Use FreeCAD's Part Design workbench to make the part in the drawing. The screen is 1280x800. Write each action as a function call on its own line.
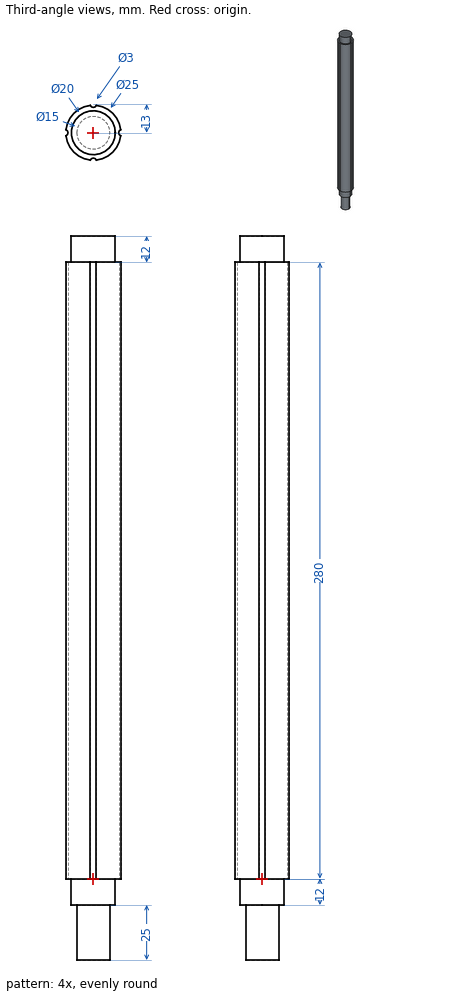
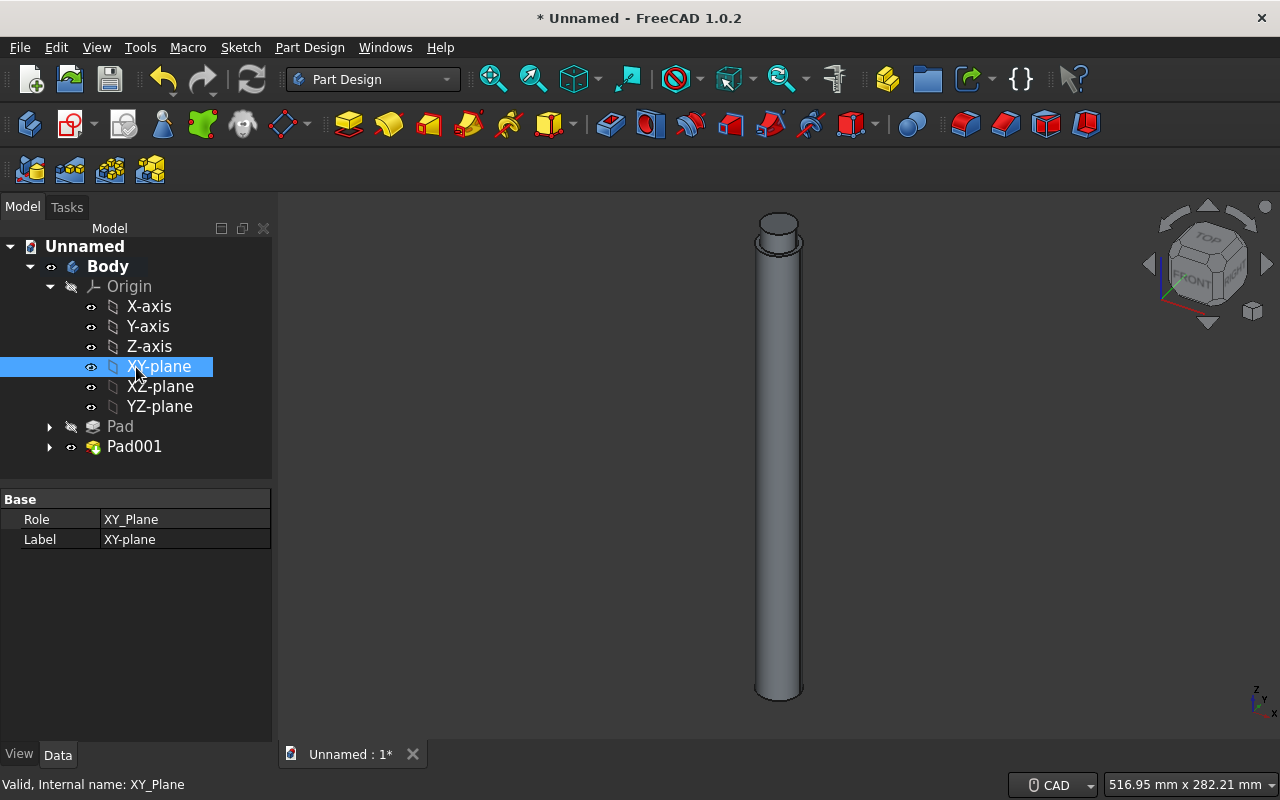
click(284, 124)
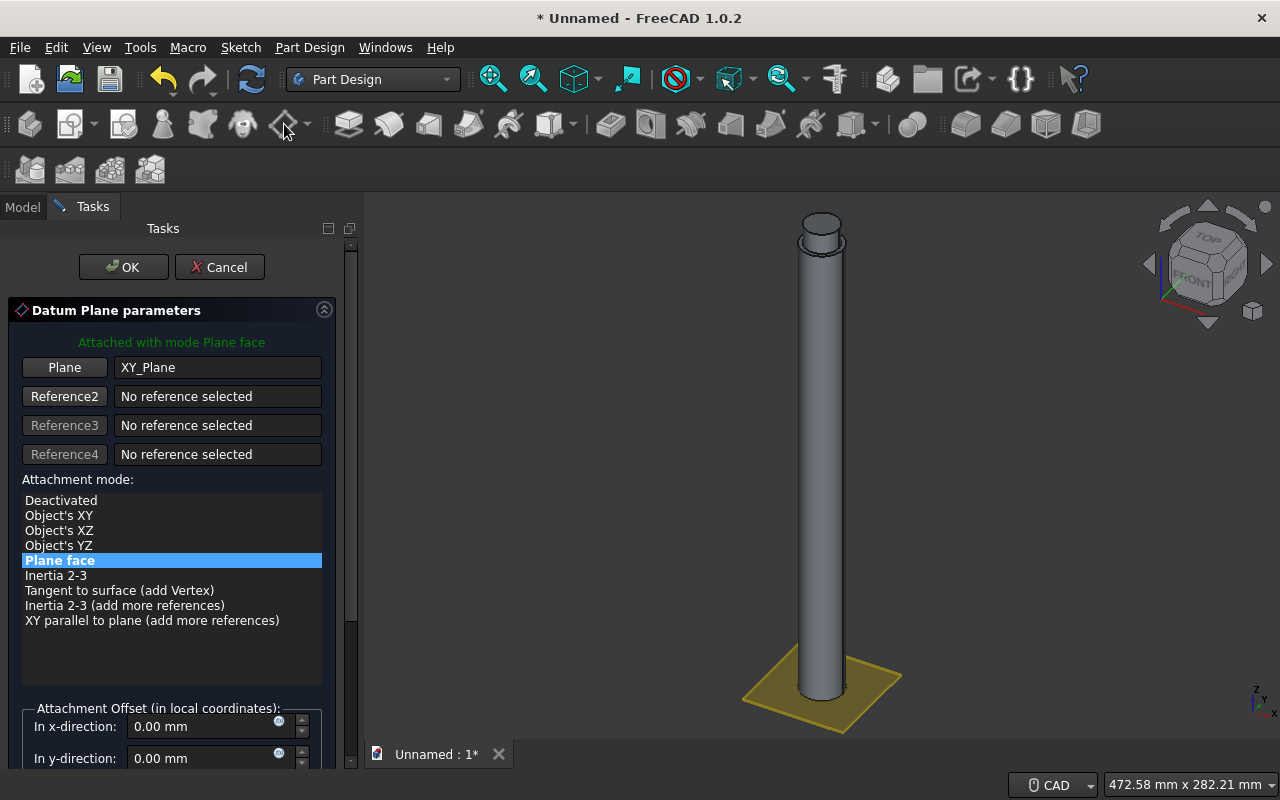
scroll(351, 503, down, 2)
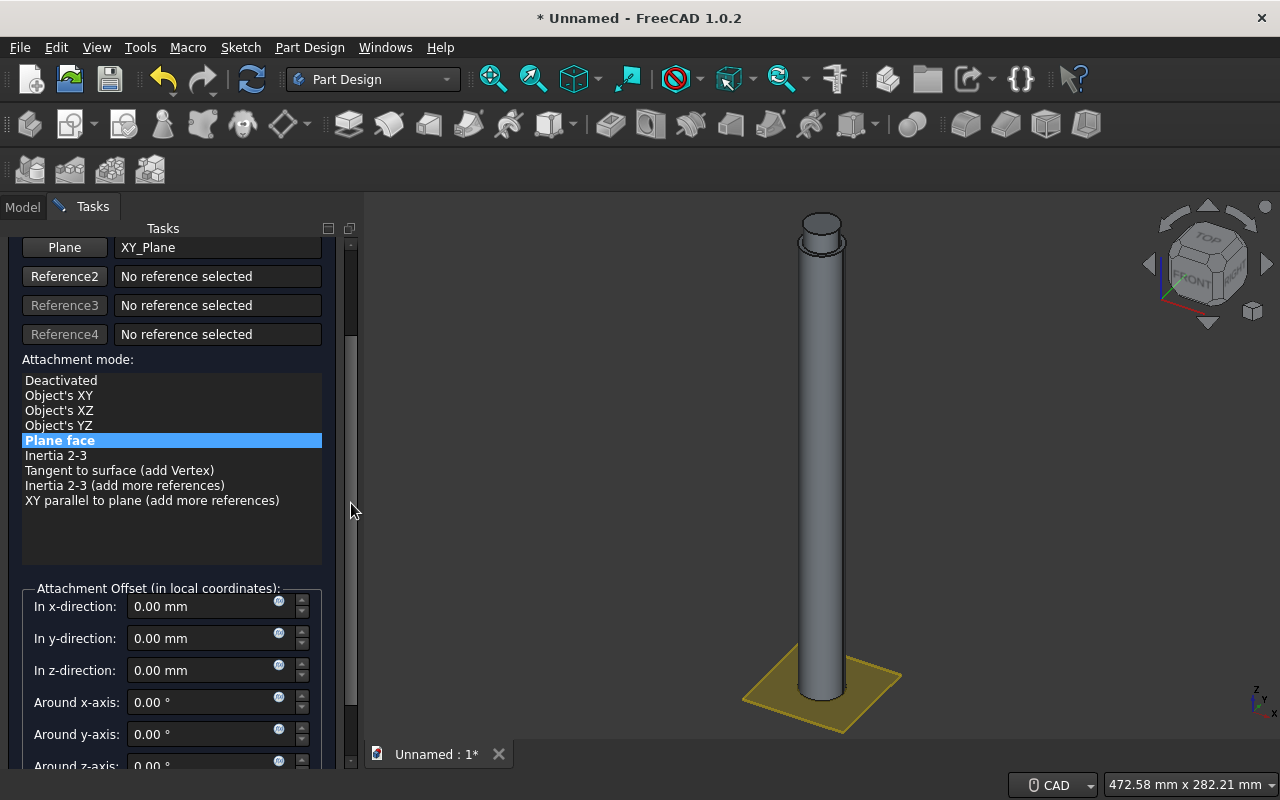
triple_click(210, 670)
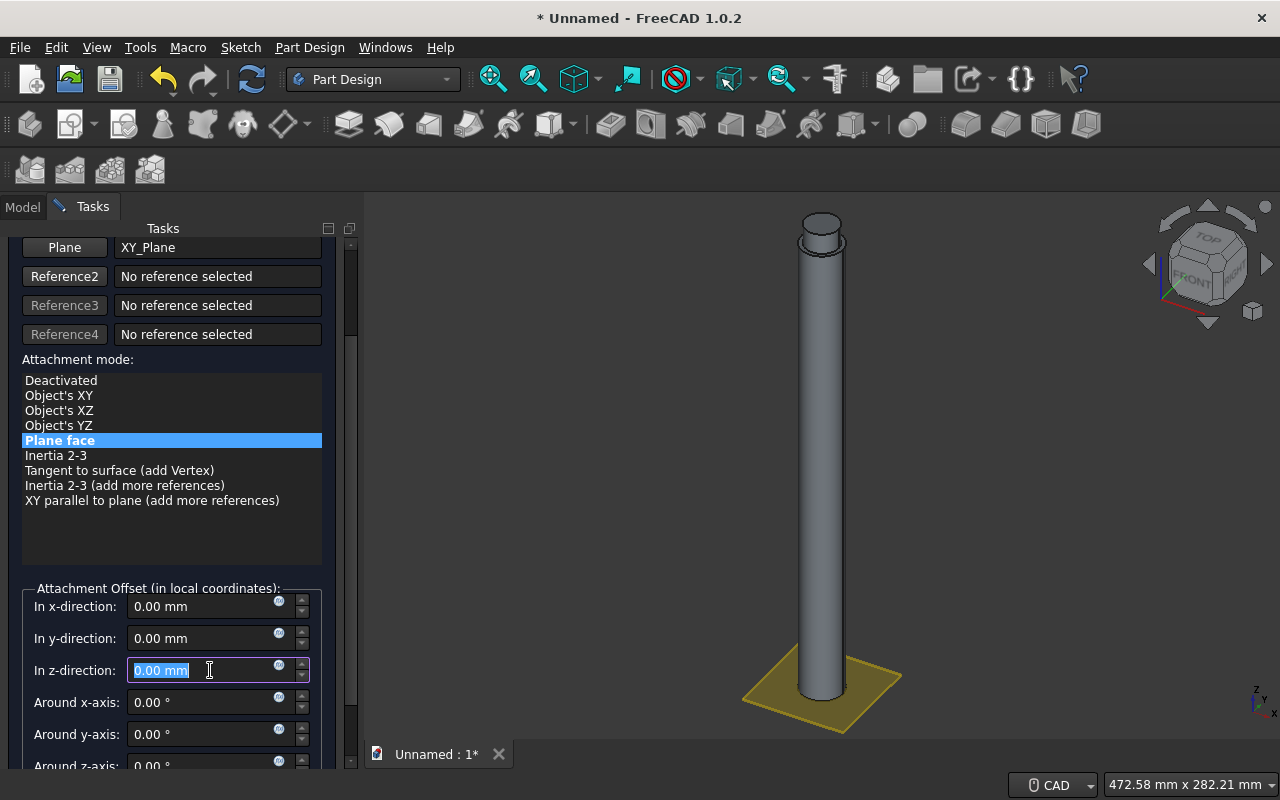
text(-12)
key(Tab)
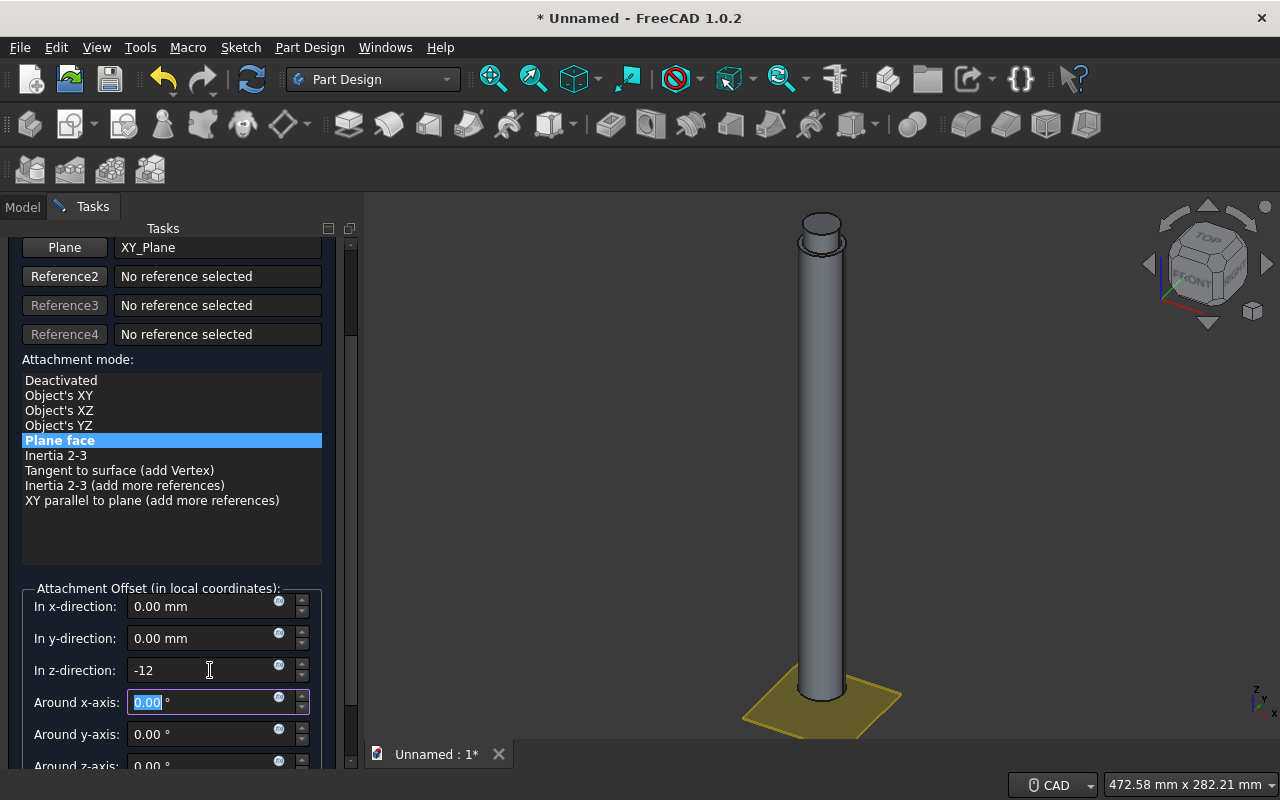
scroll(351, 503, up, 3)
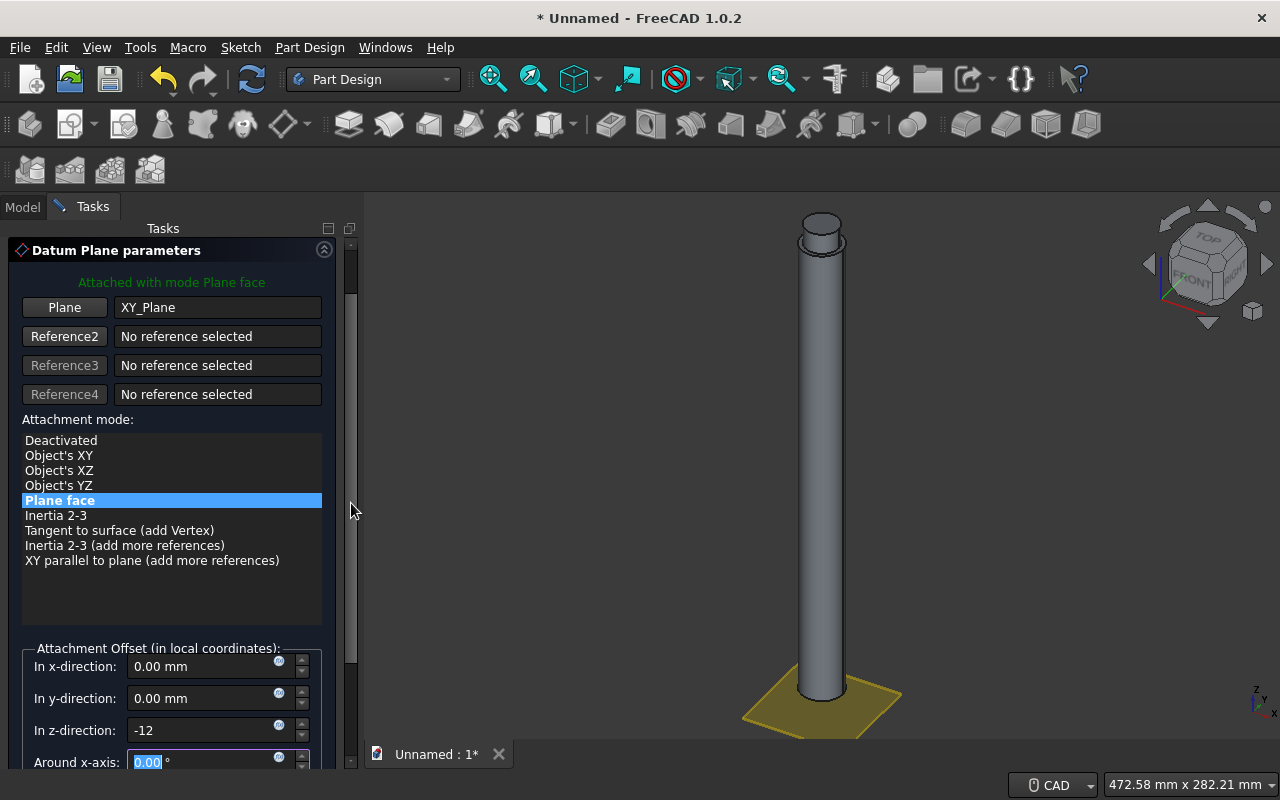
click(124, 267)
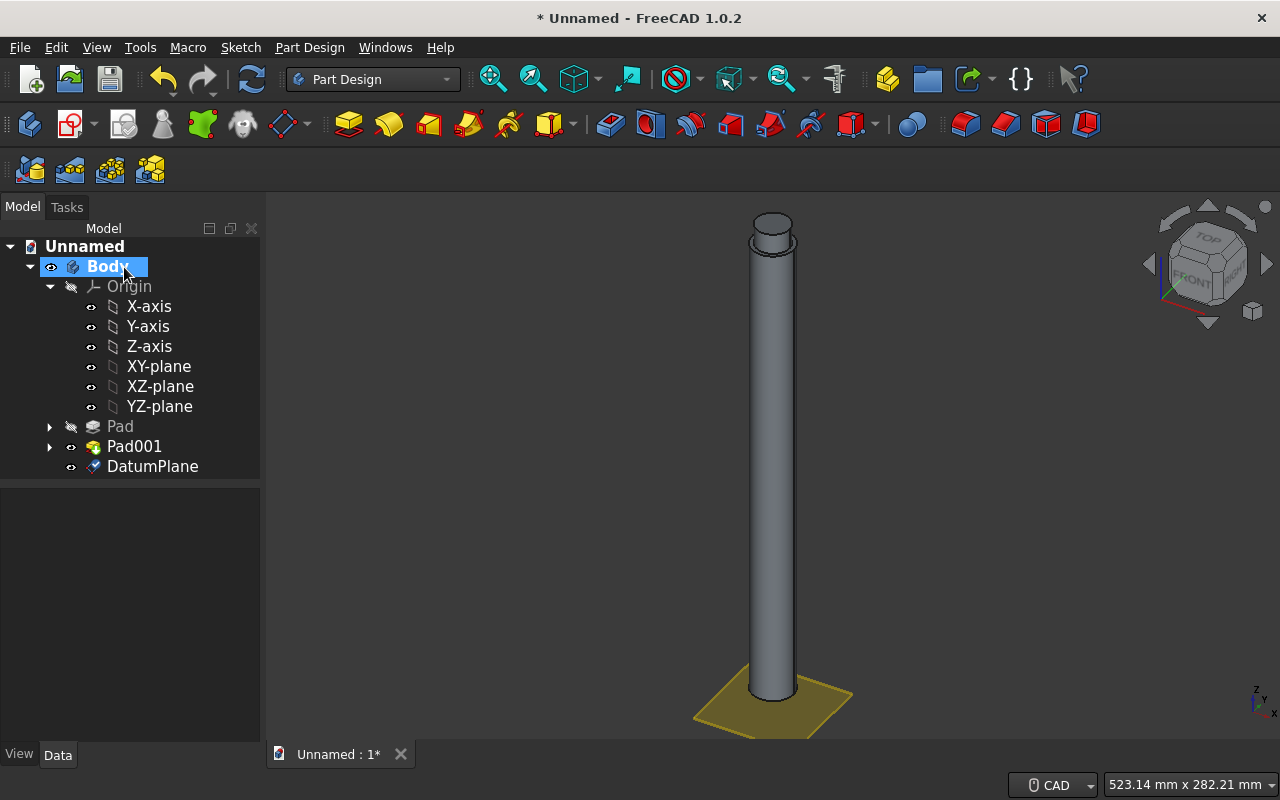
click(116, 467)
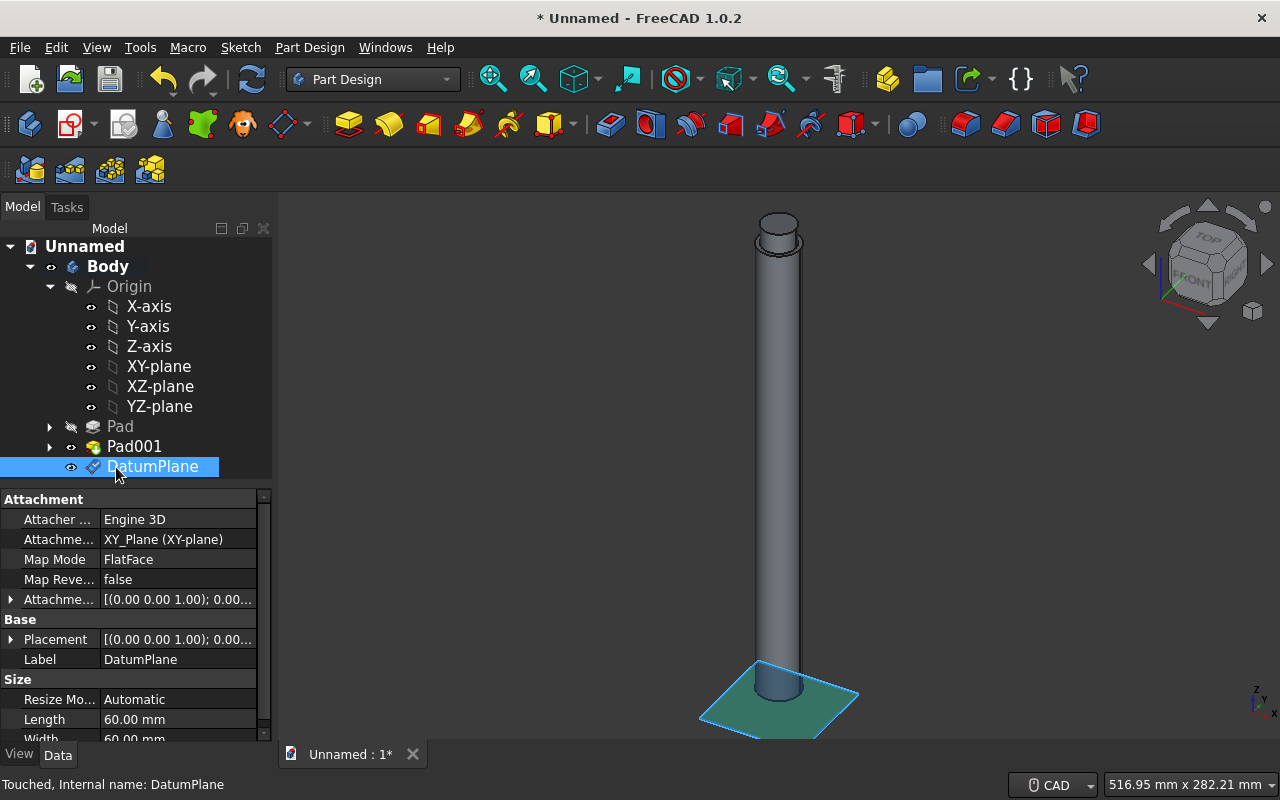
click(70, 124)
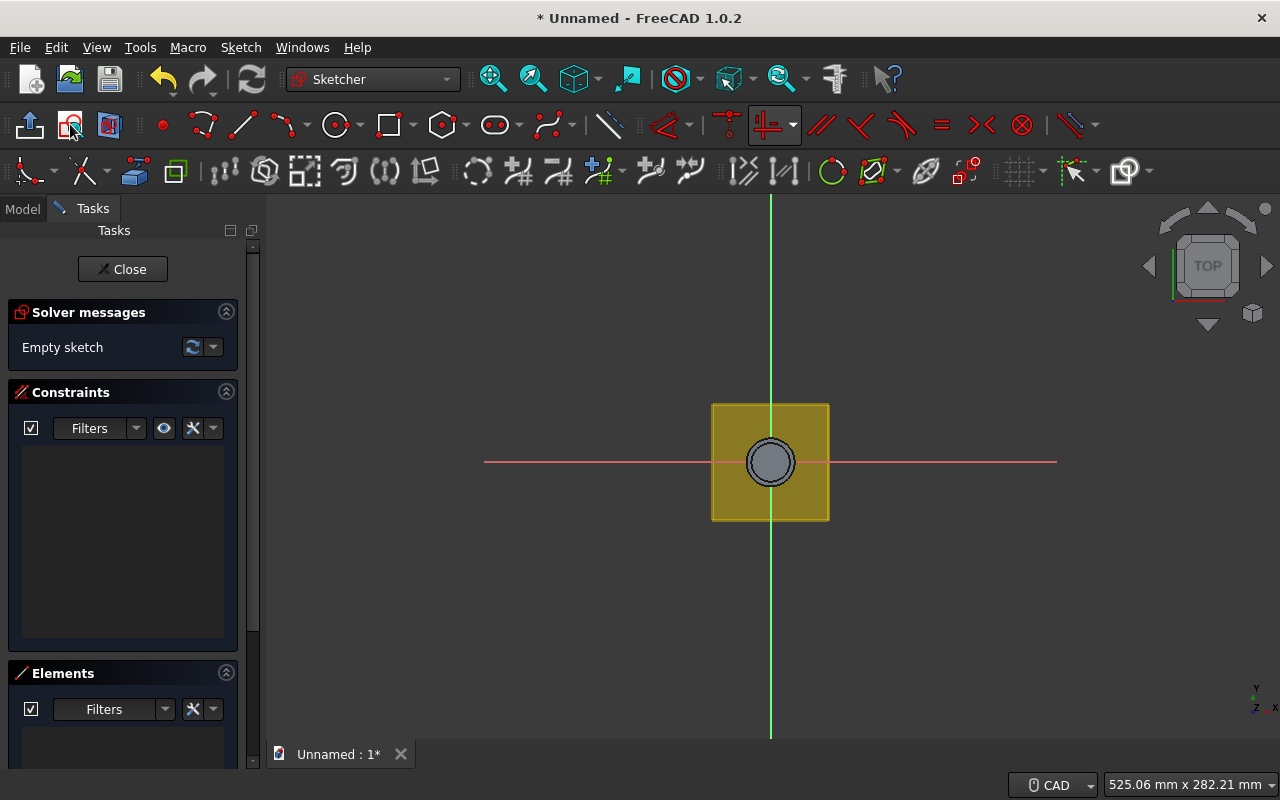
key(q)
key(s)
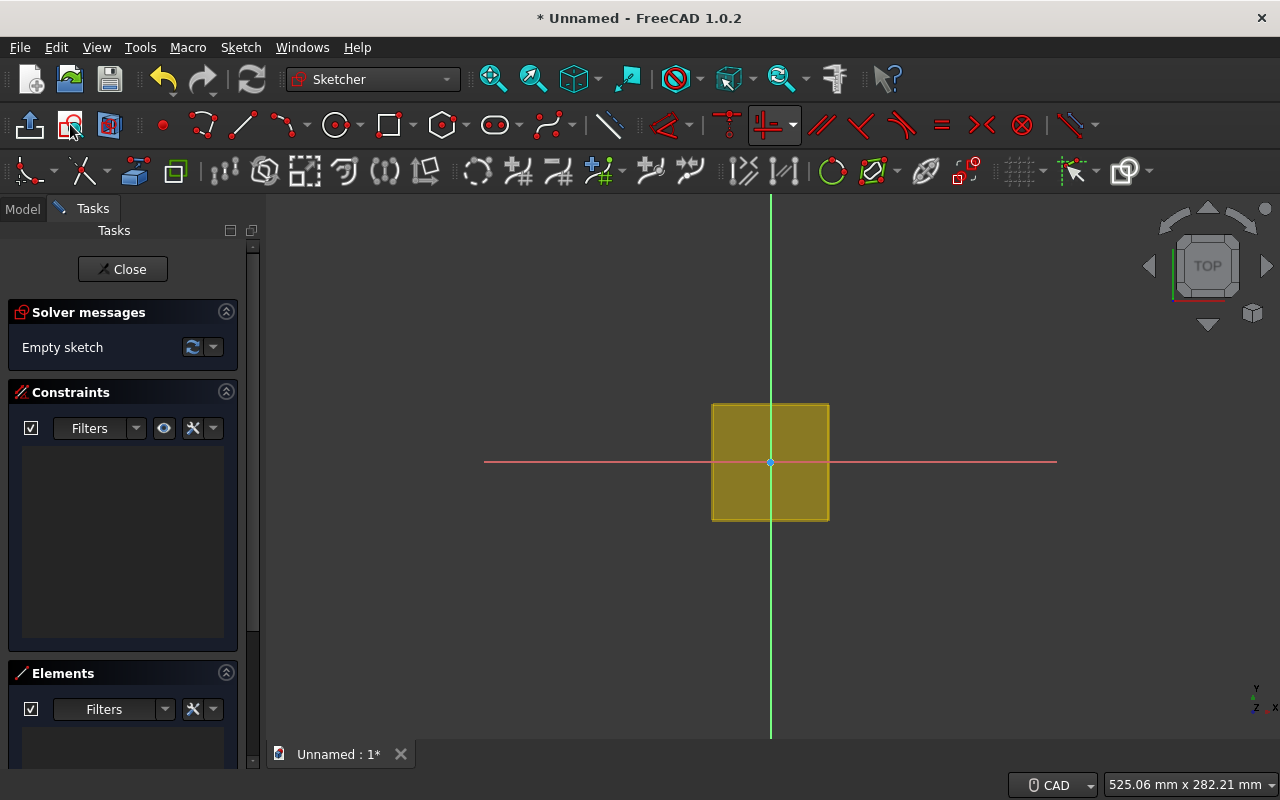
scroll(779, 462, up, 11)